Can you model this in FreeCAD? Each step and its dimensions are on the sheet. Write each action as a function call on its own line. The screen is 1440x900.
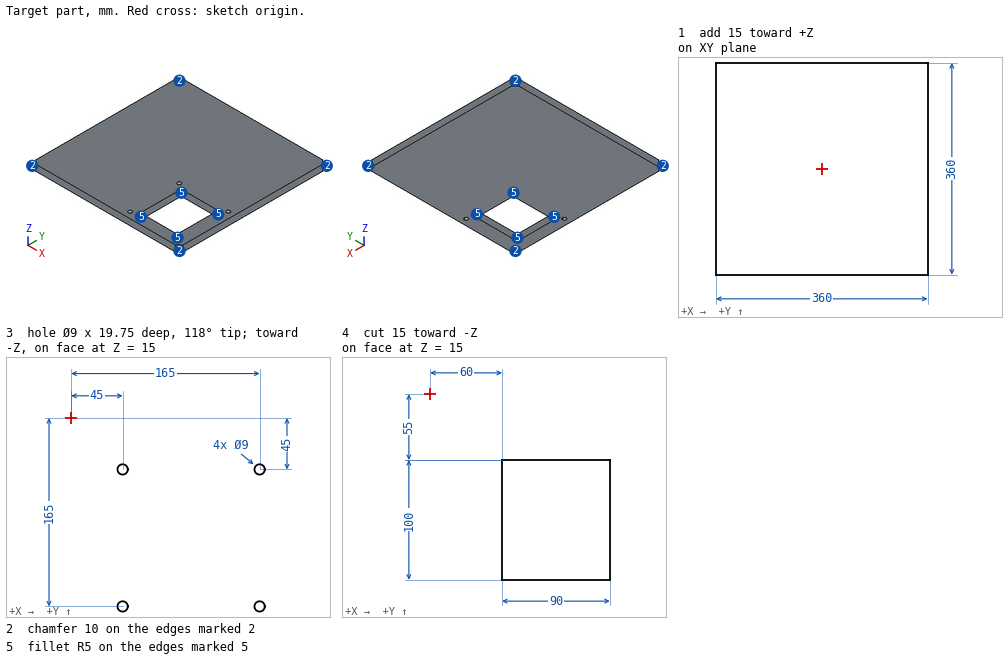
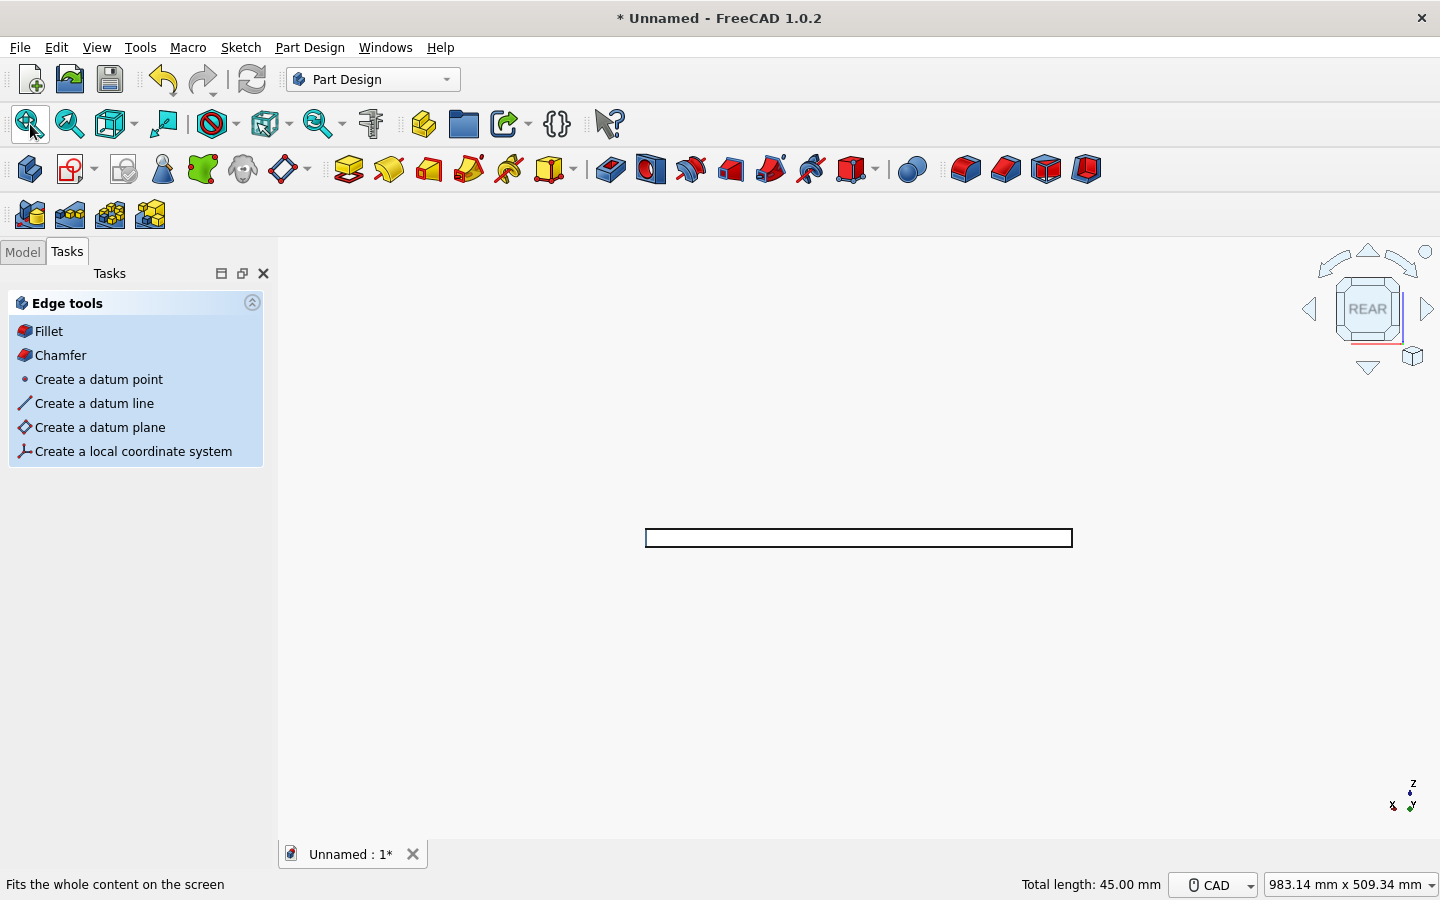
click(30, 124)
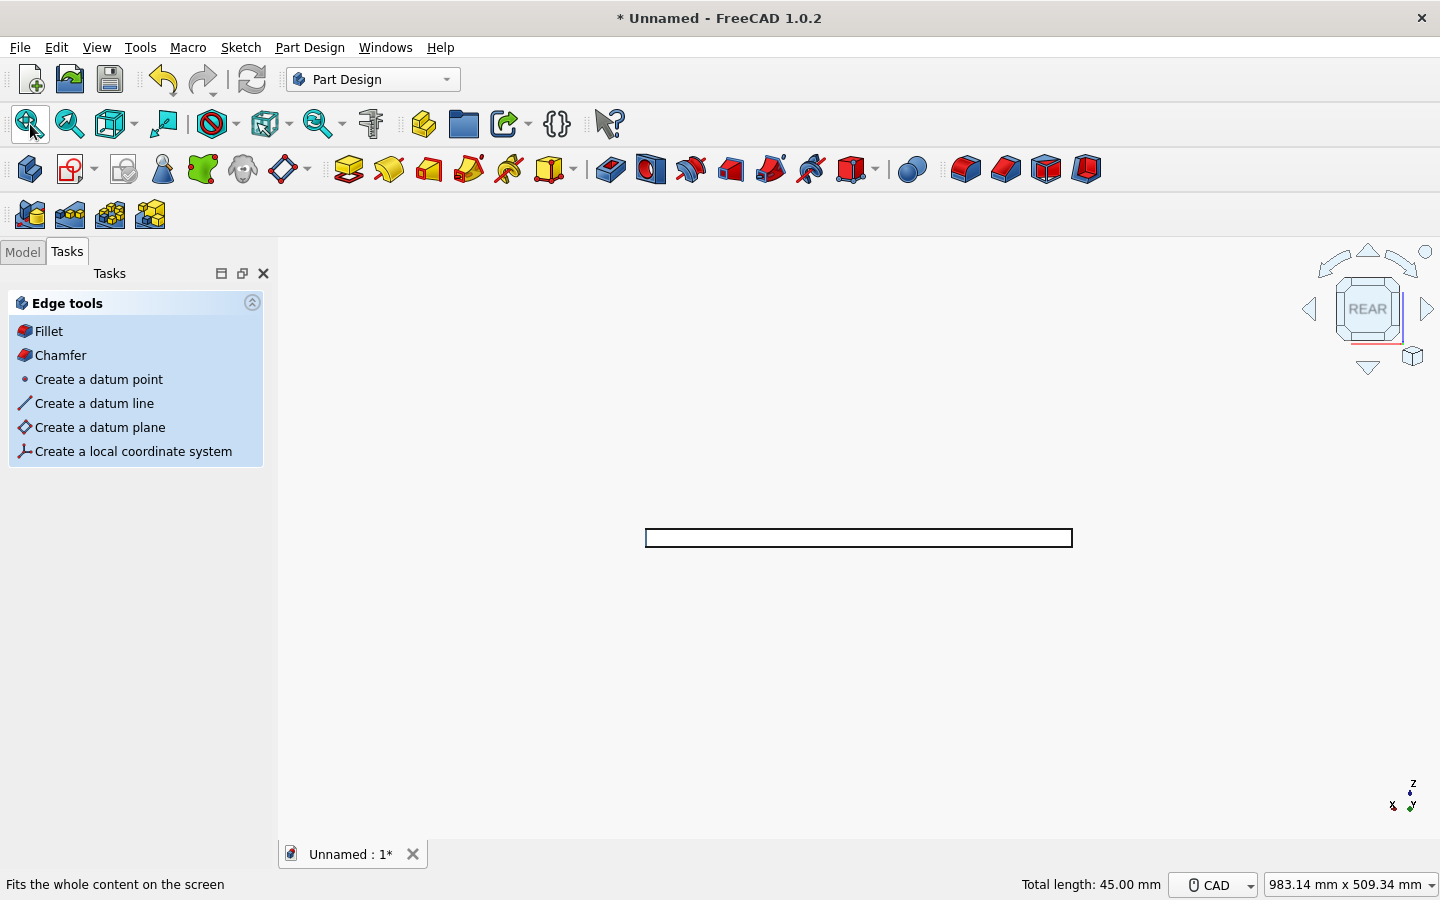
click(1072, 537, ctrl)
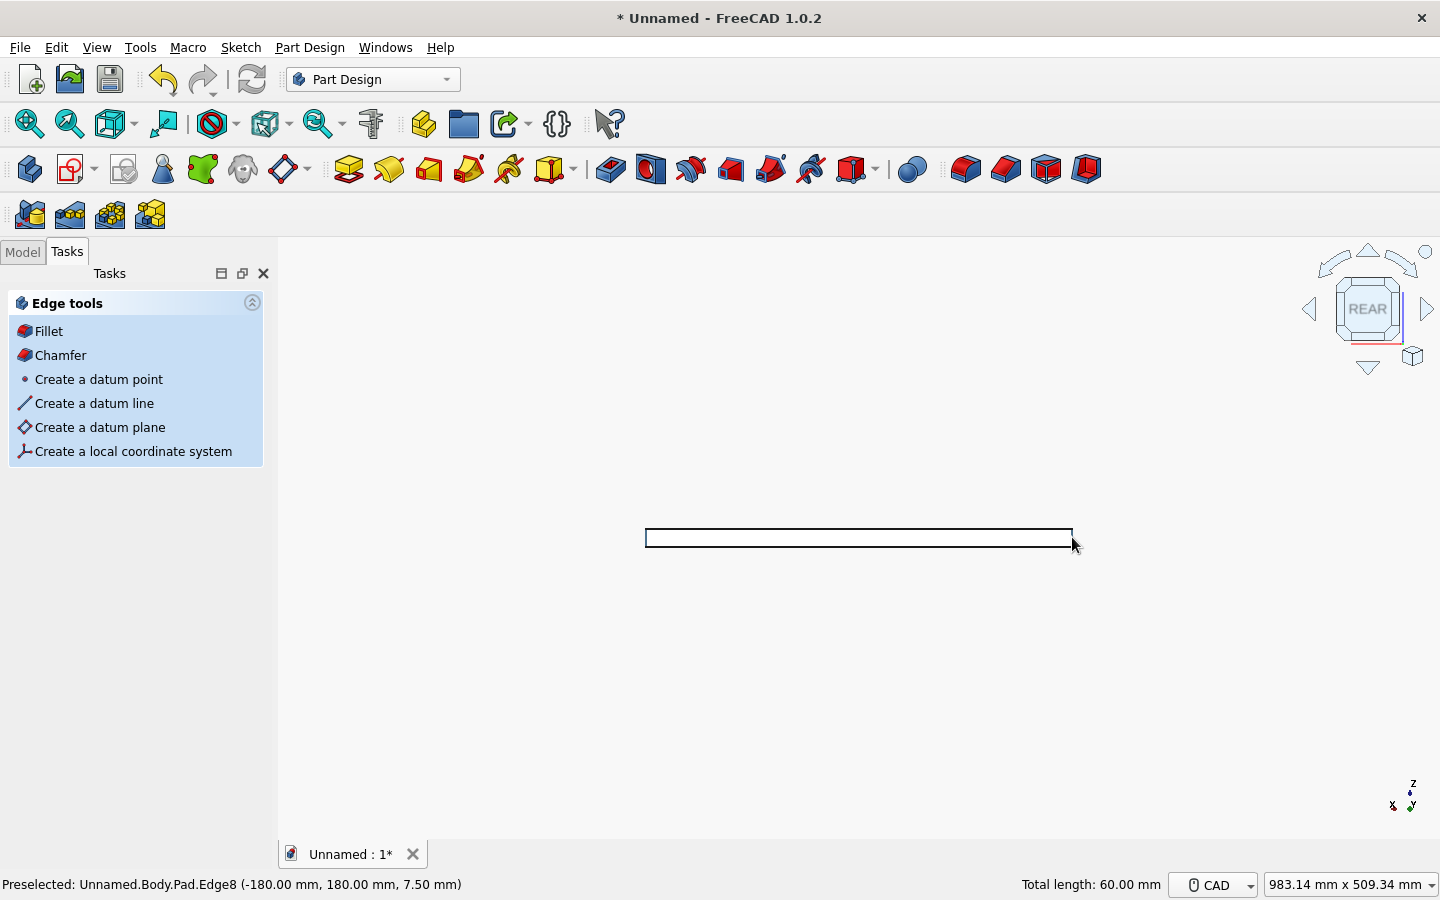
click(1006, 170)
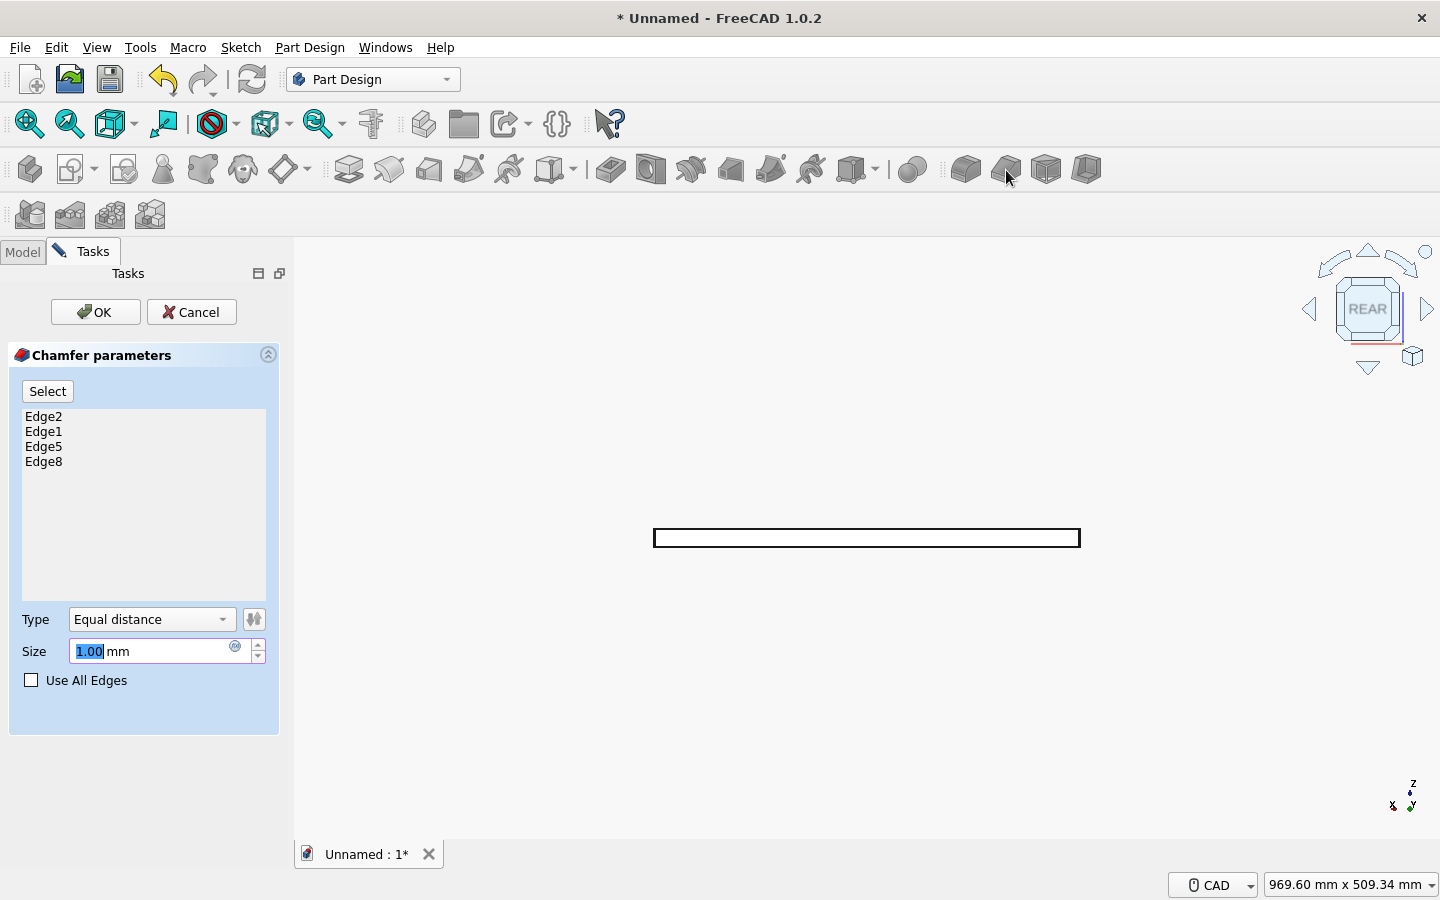
text(10)
key(Tab)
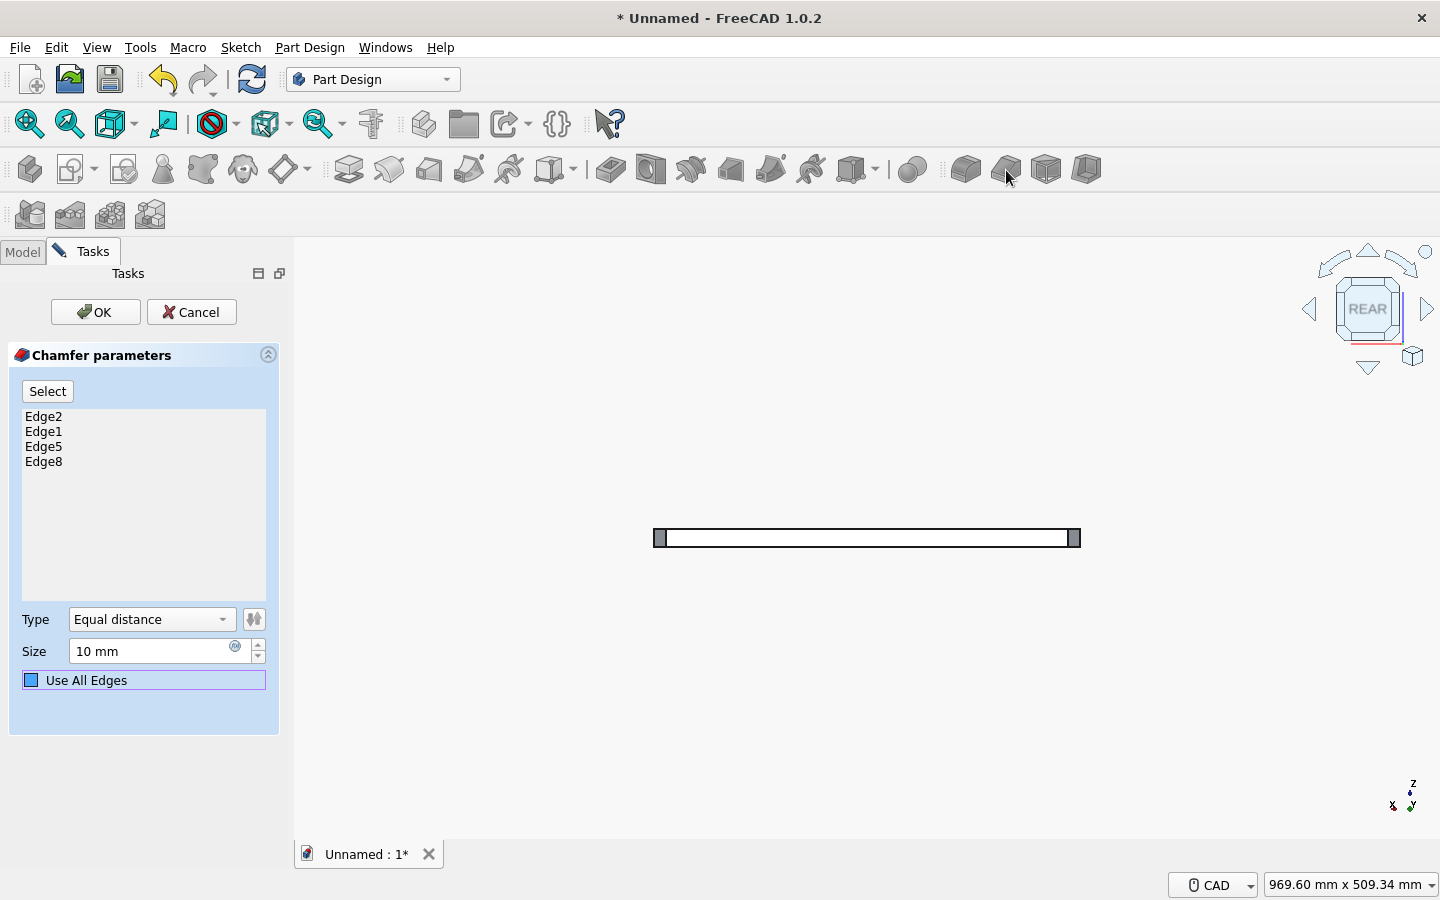
click(96, 312)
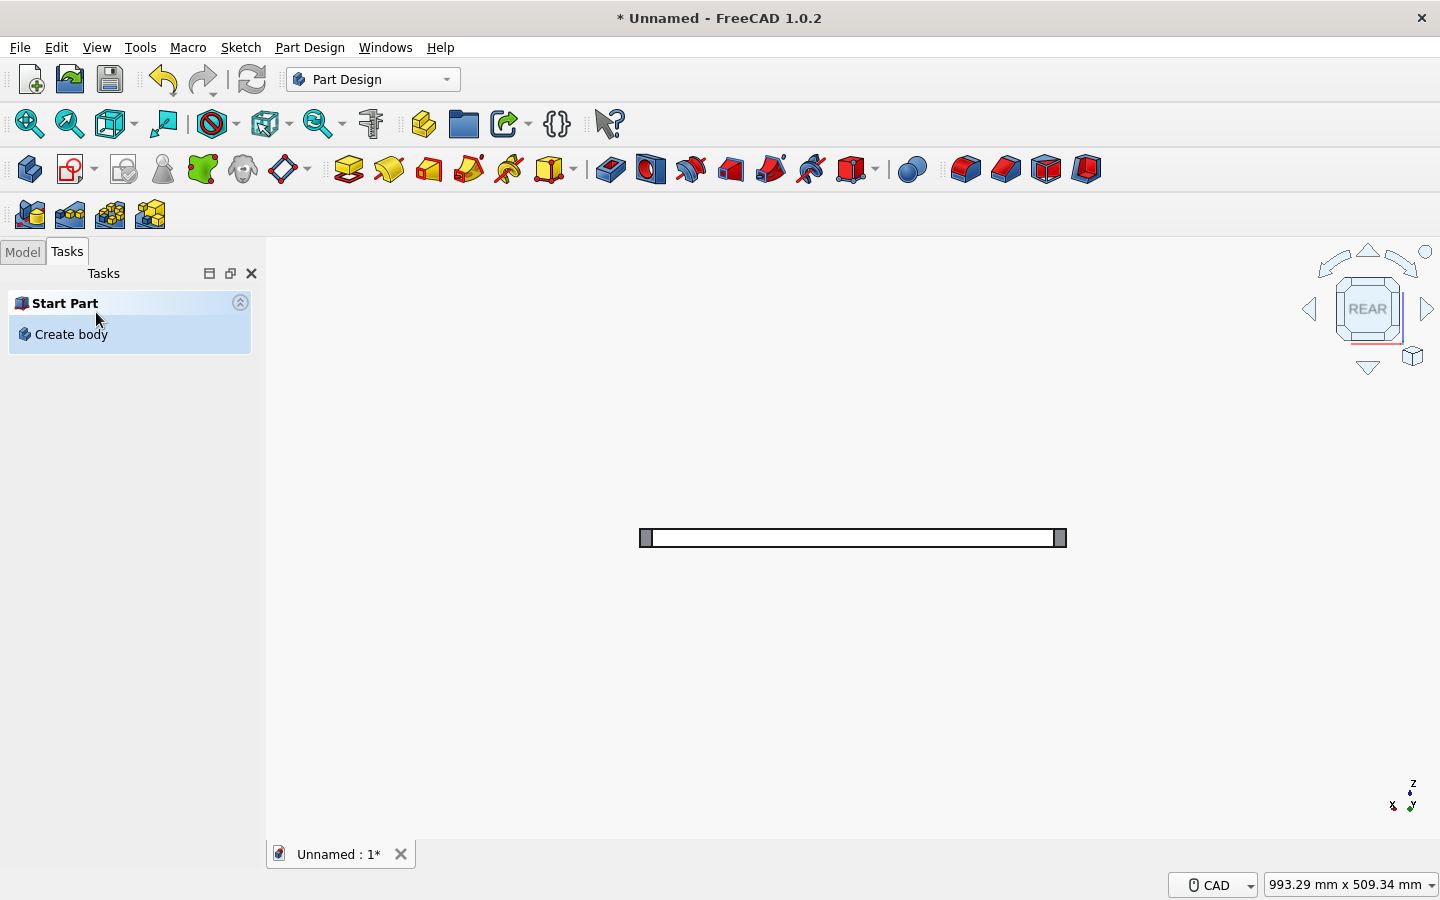
key(v)
key(f)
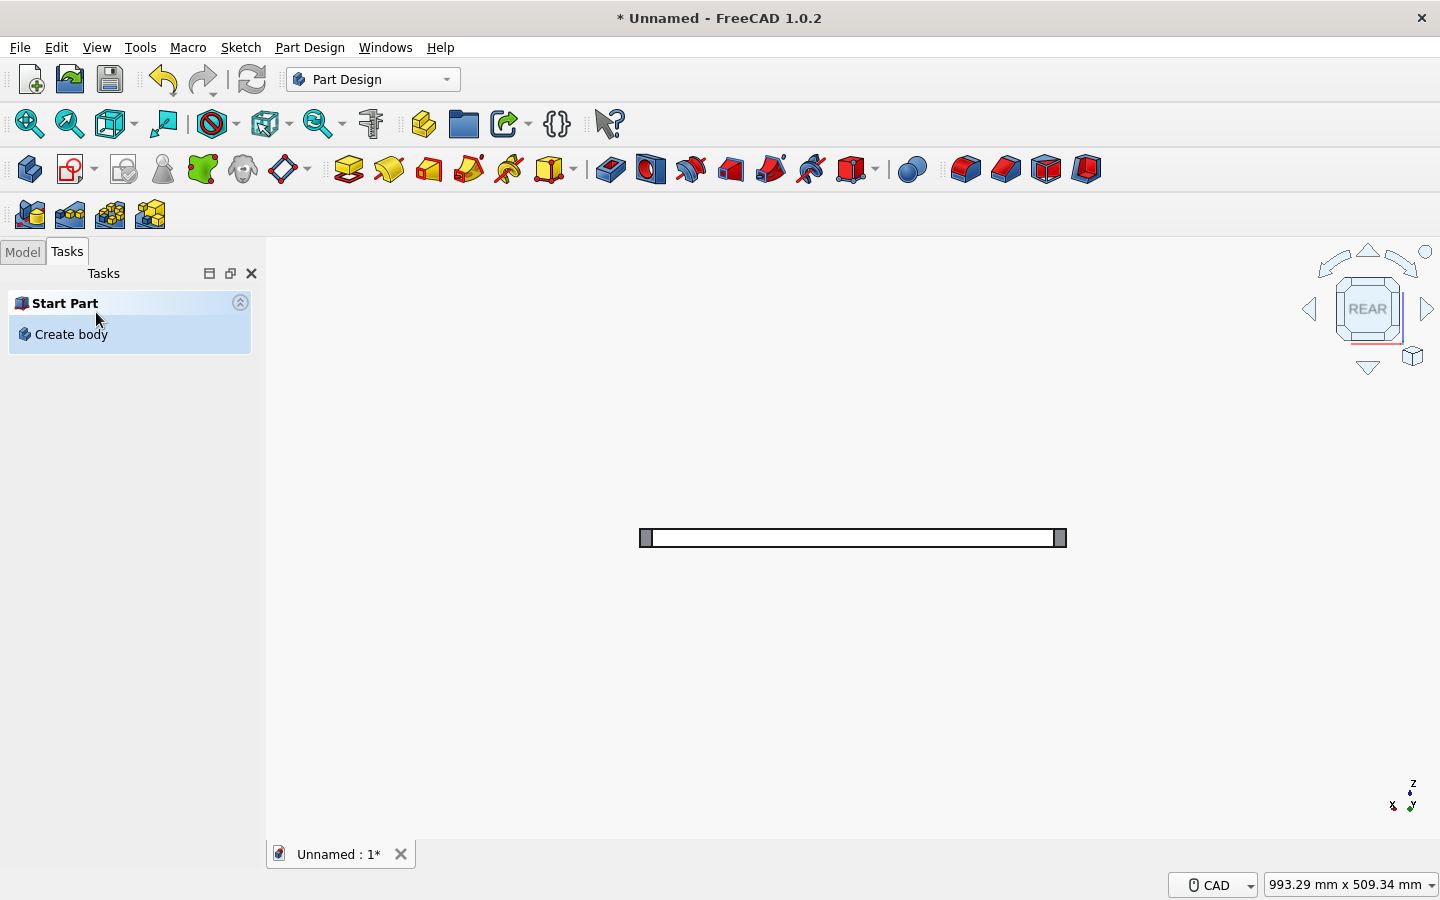
key(0)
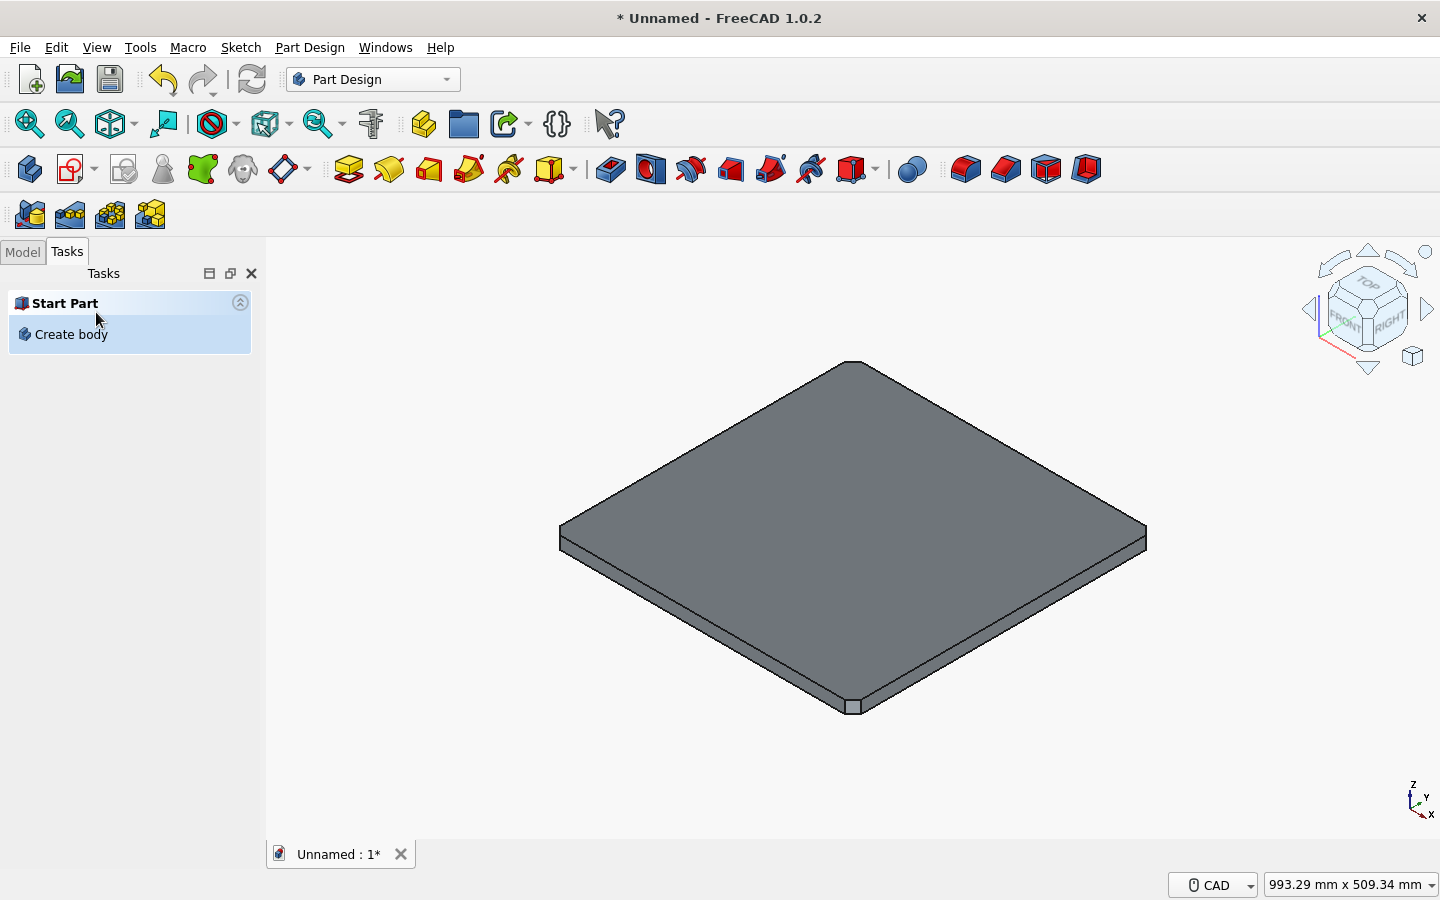
click(853, 530)